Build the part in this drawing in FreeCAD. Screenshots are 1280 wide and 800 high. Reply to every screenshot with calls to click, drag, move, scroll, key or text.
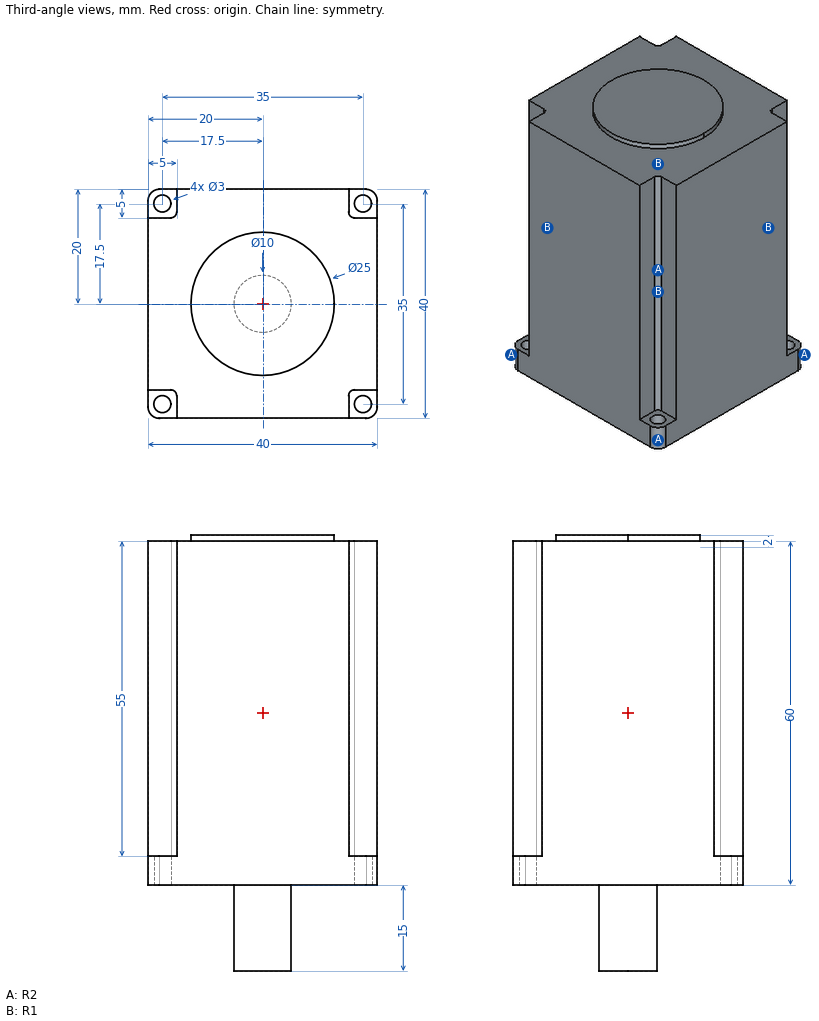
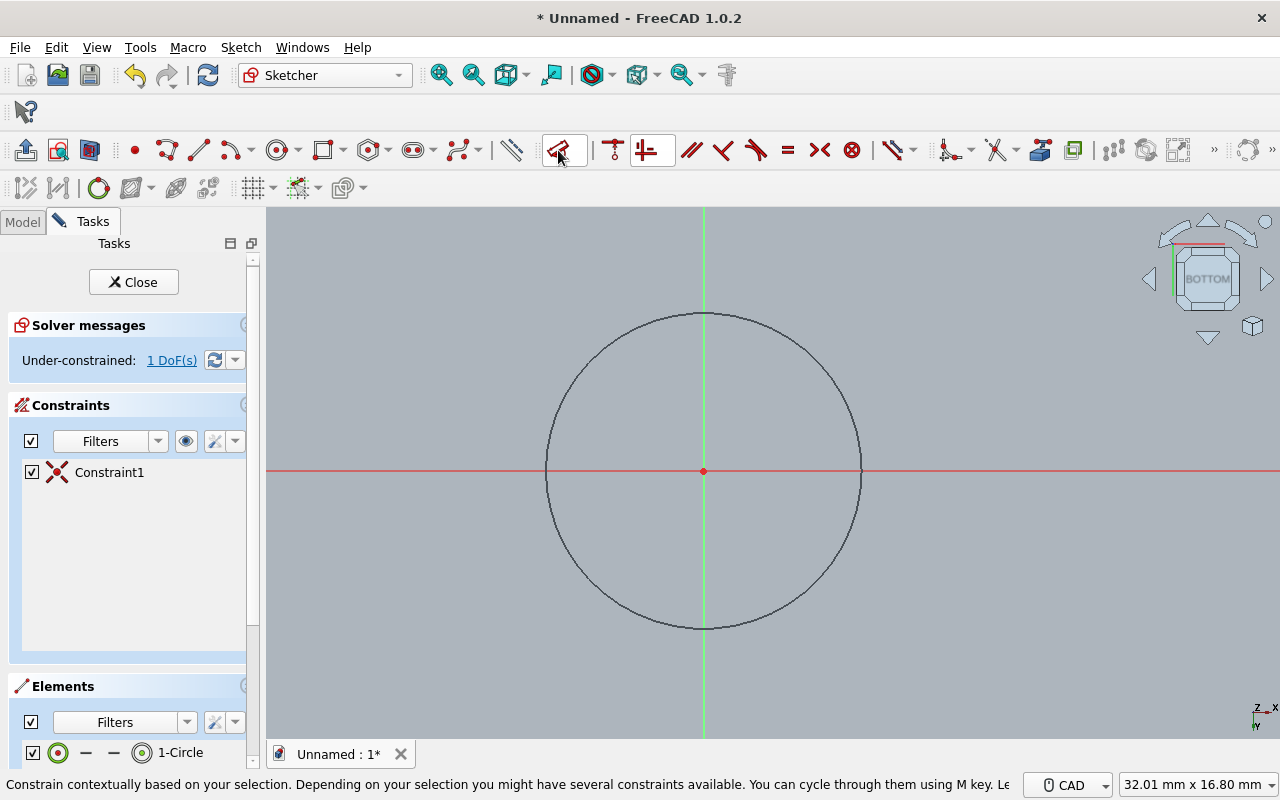
click(815, 359)
click(838, 336)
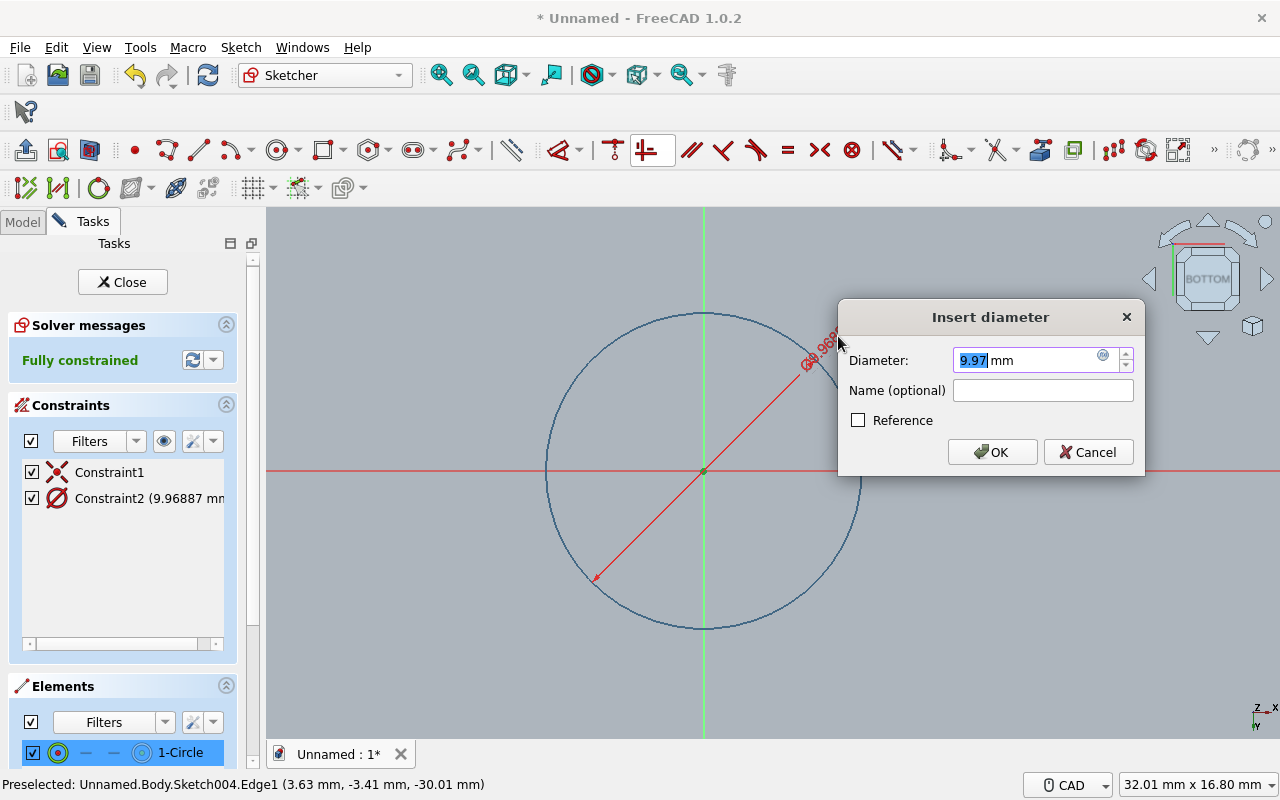
text(10)
key(Return)
key(Escape)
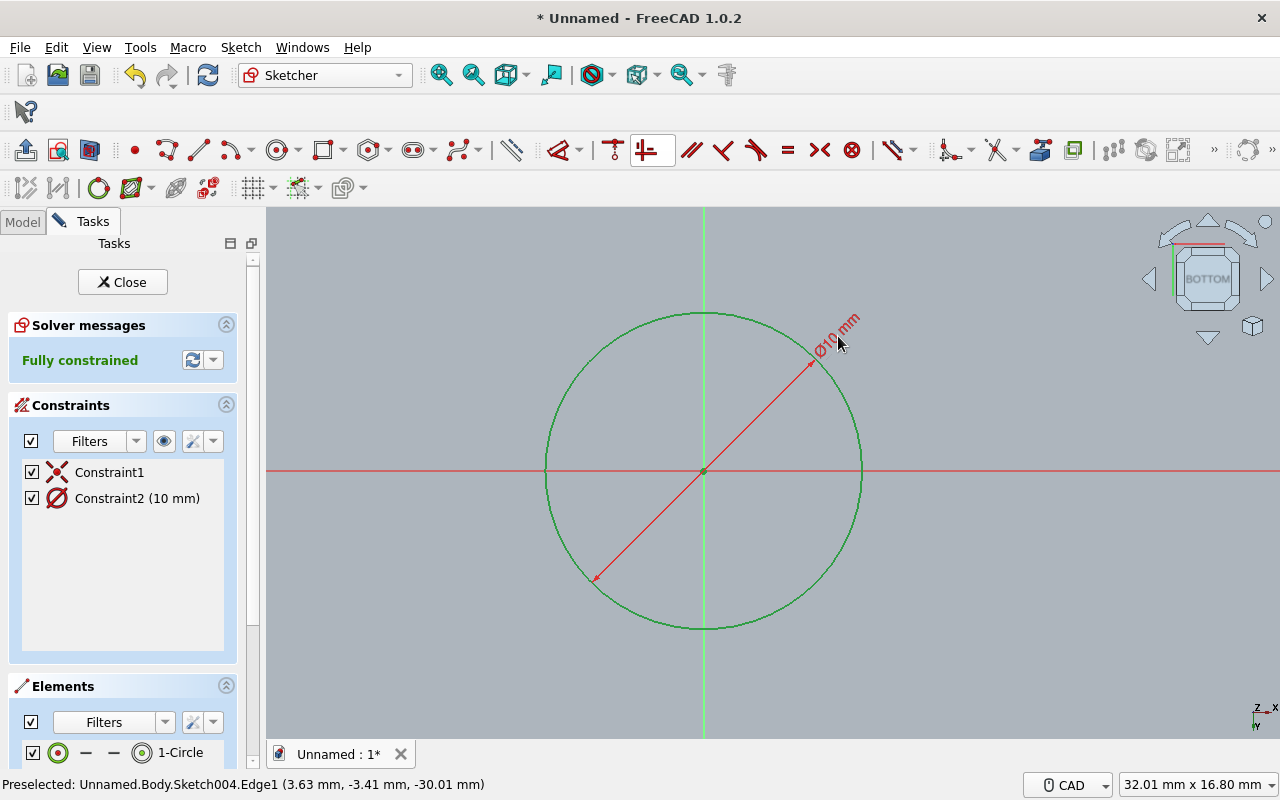
click(123, 282)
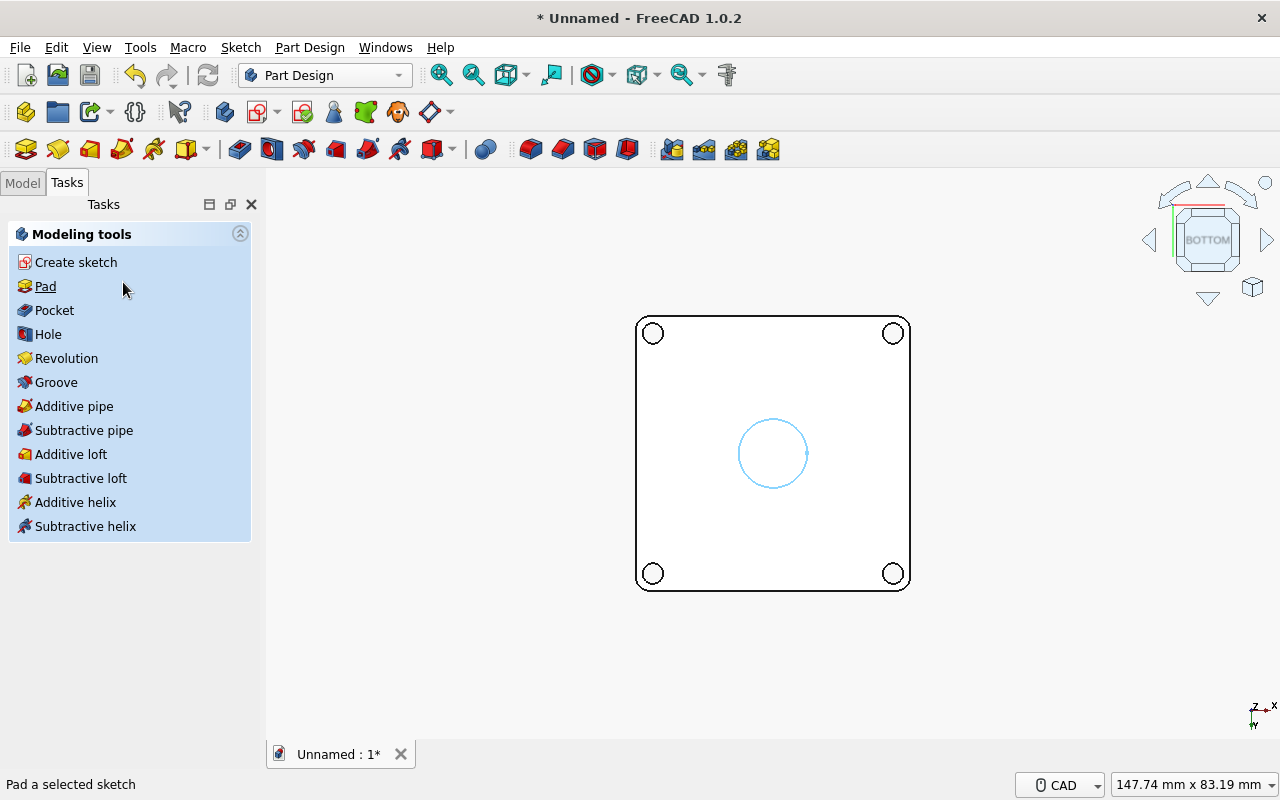
click(26, 150)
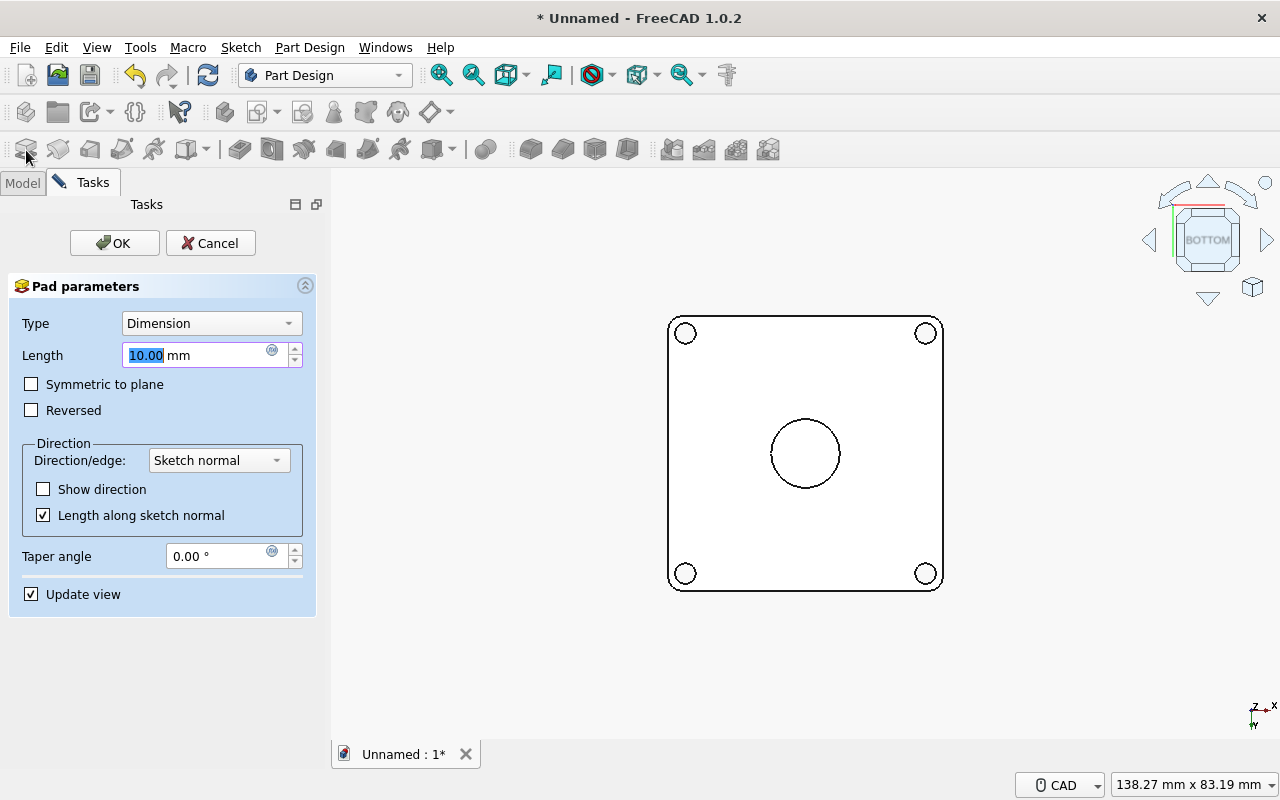
text(15)
key(Tab)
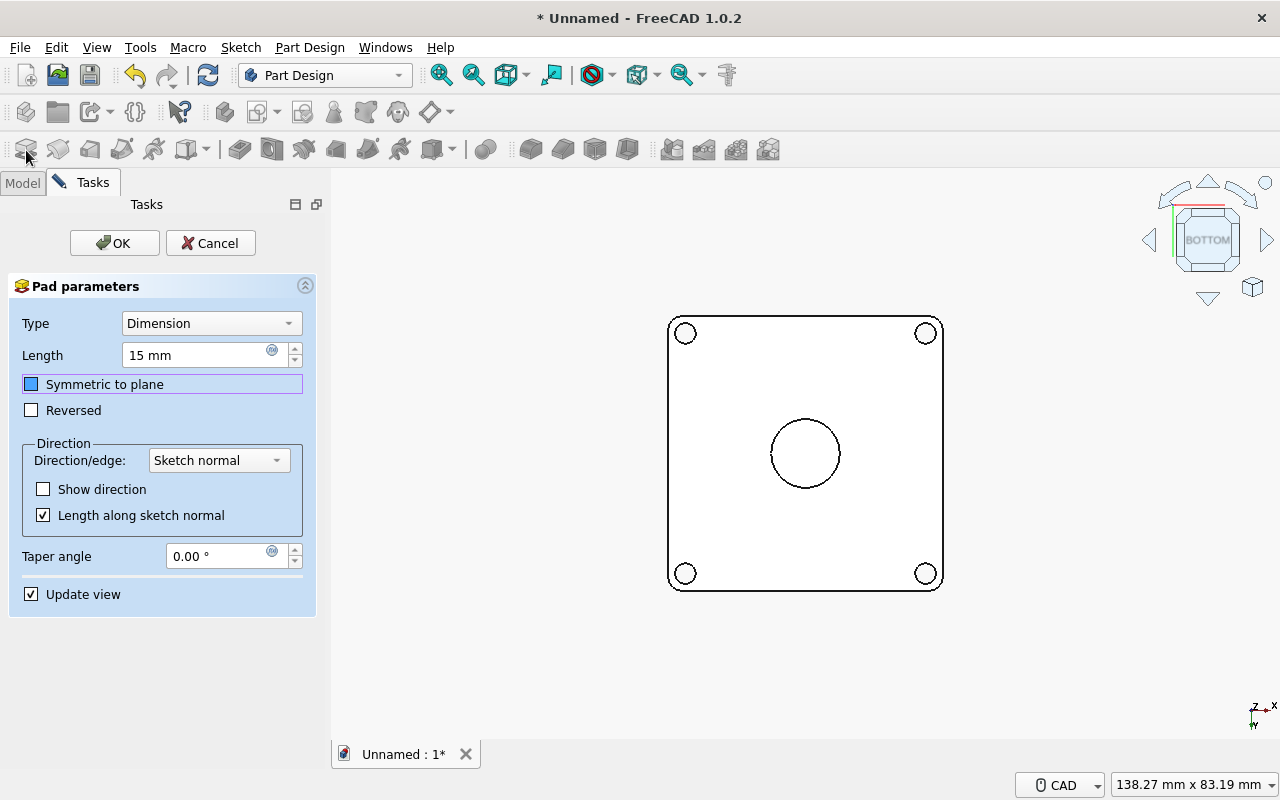
click(115, 243)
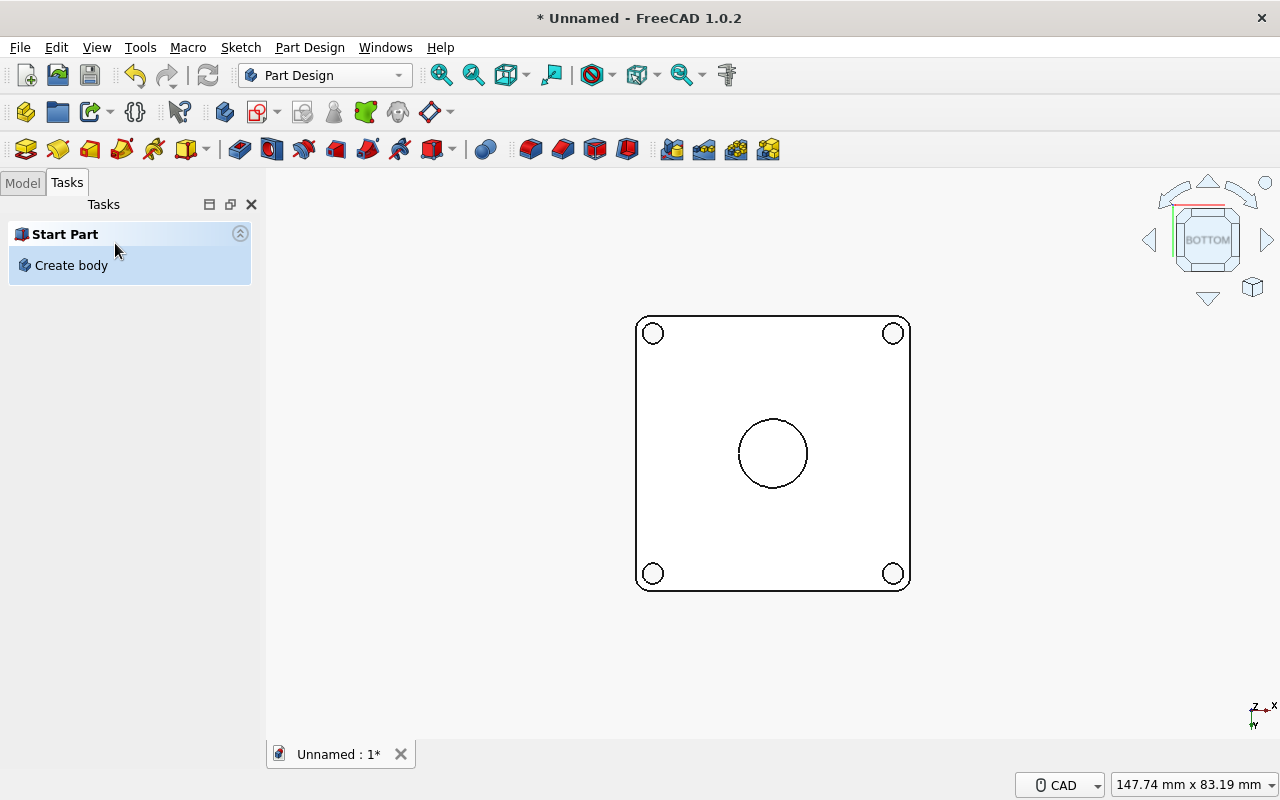
key(0)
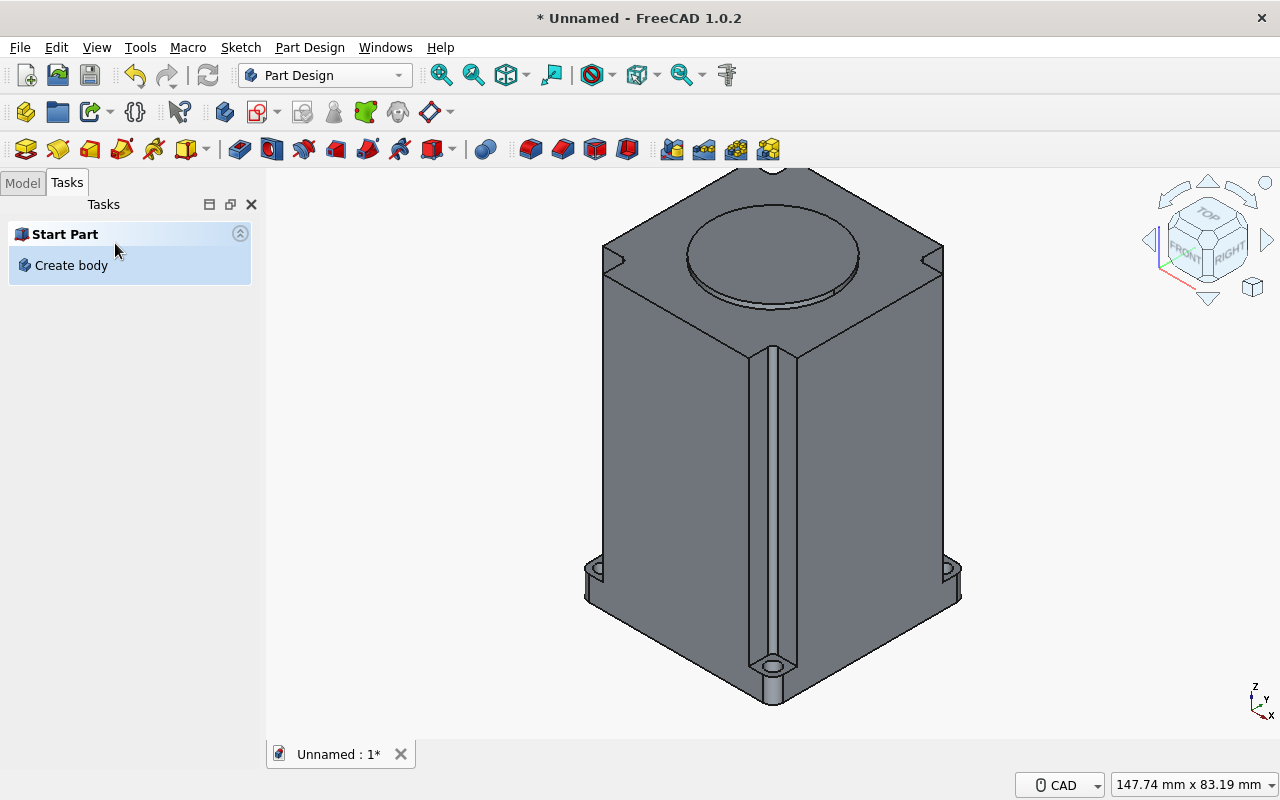
click(442, 76)